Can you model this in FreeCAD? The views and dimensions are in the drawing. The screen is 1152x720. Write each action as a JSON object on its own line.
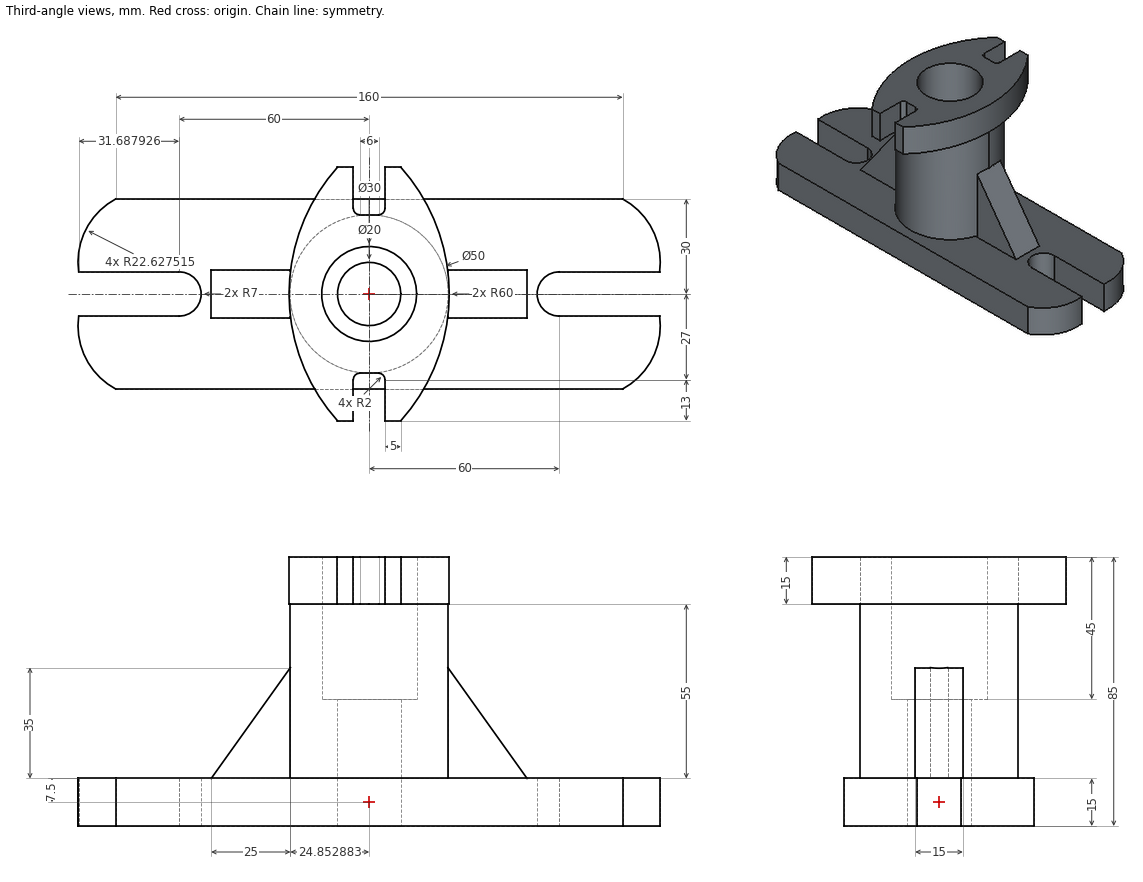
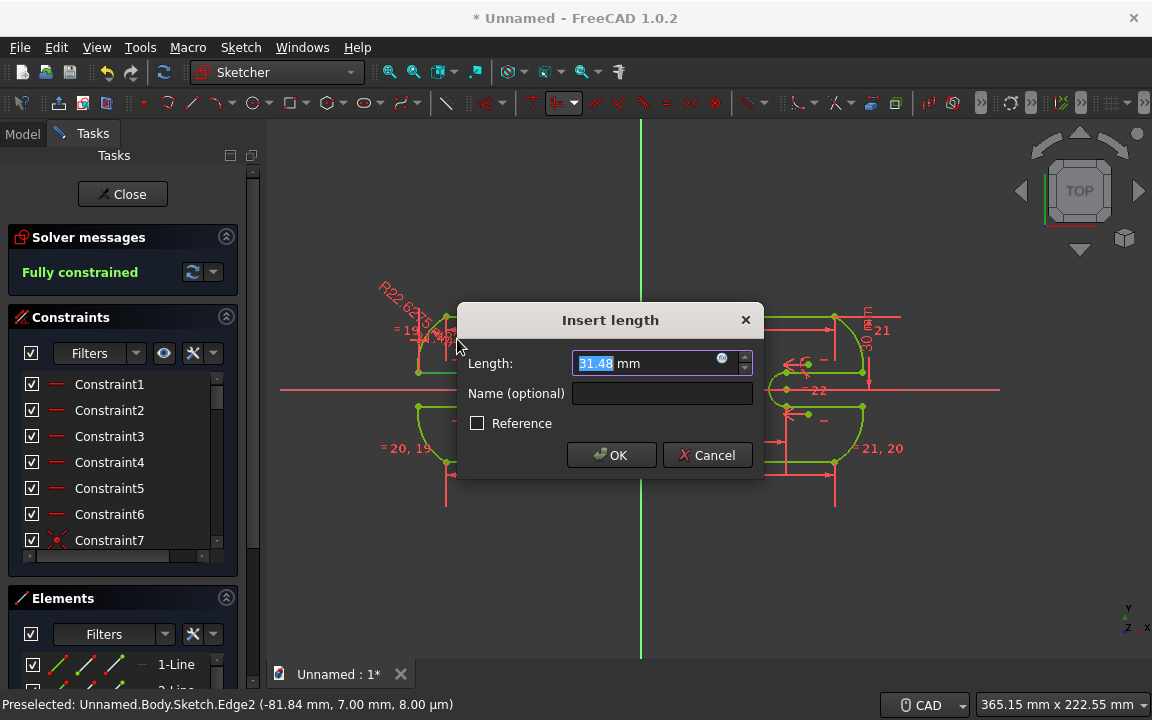
{"action": "type", "text": "31.687926"}
{"action": "key", "text": "Return"}
{"action": "key", "text": "Escape"}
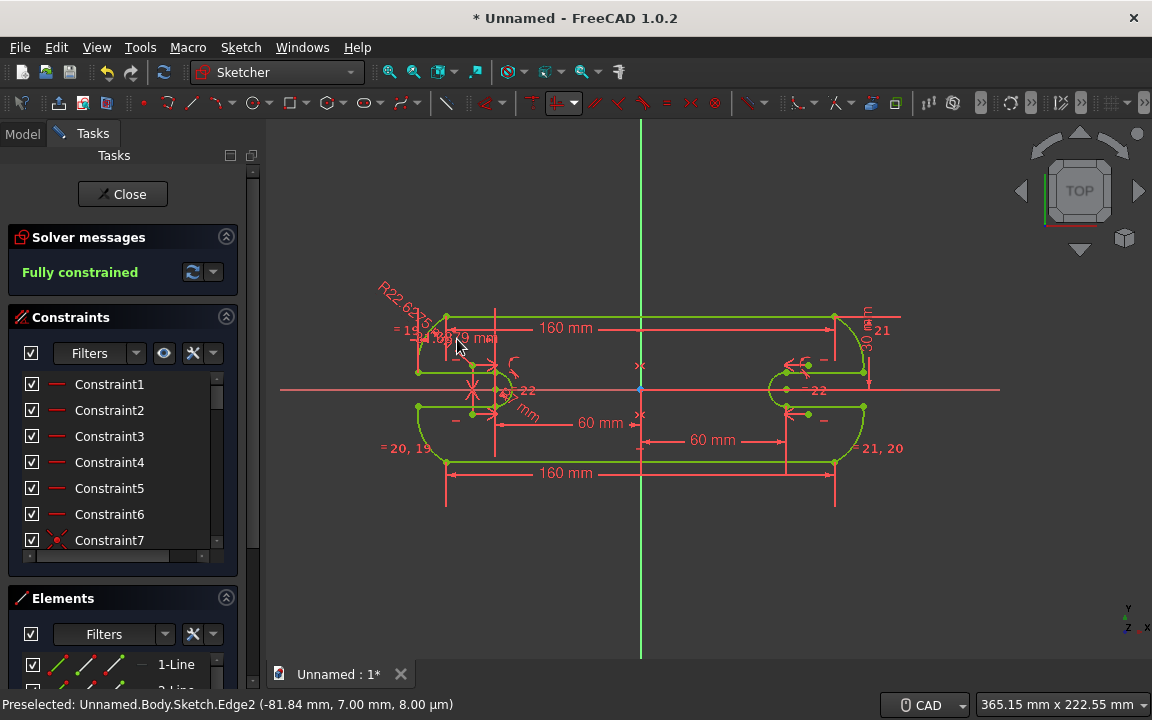
{"action": "left_click", "coordinate": [123, 194]}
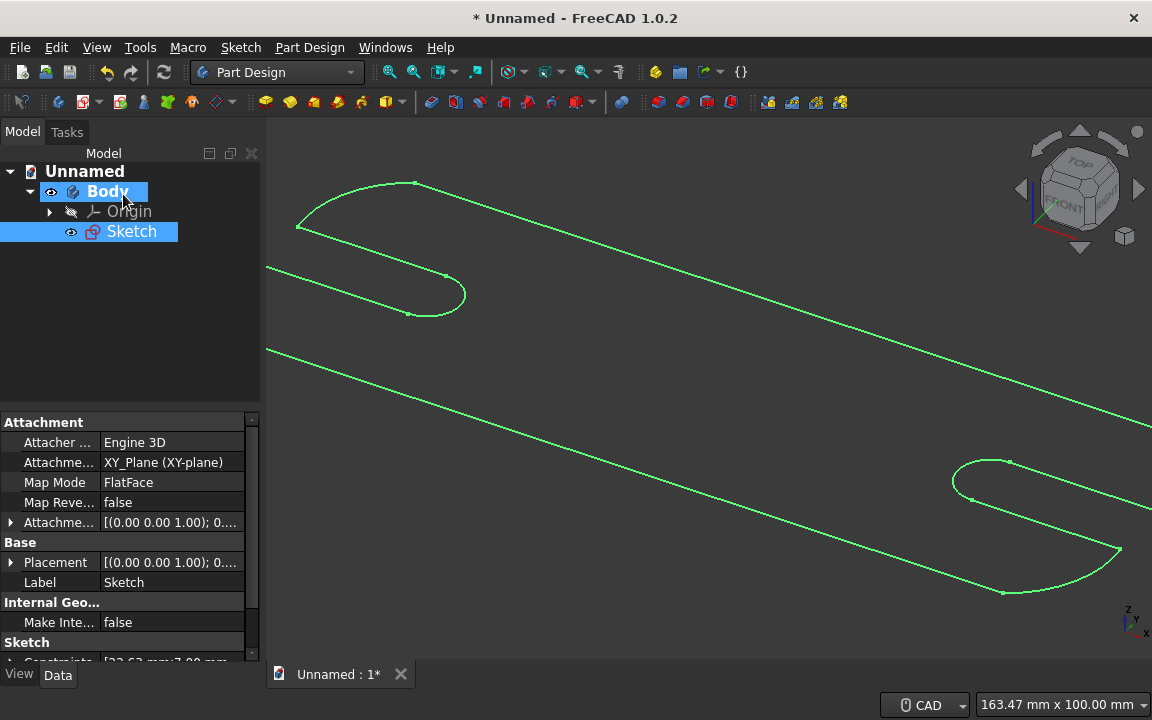
{"action": "left_click", "coordinate": [266, 102]}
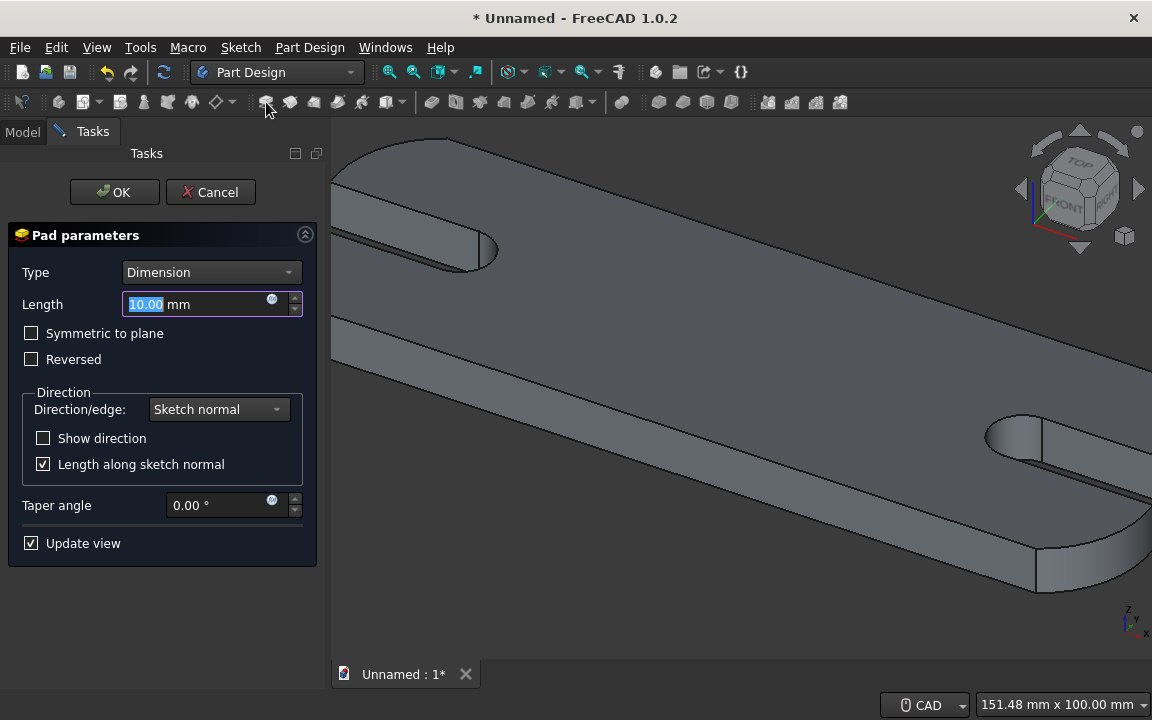
{"action": "type", "text": "15"}
{"action": "key", "text": "Tab"}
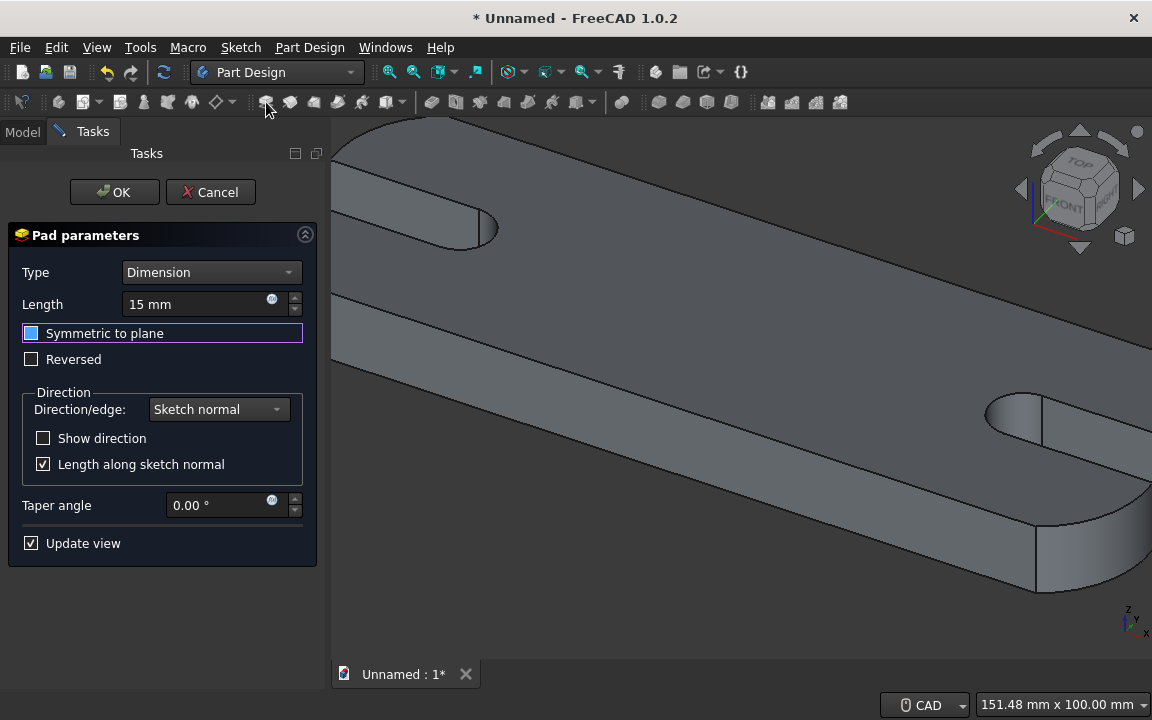
{"action": "left_click", "coordinate": [30, 333]}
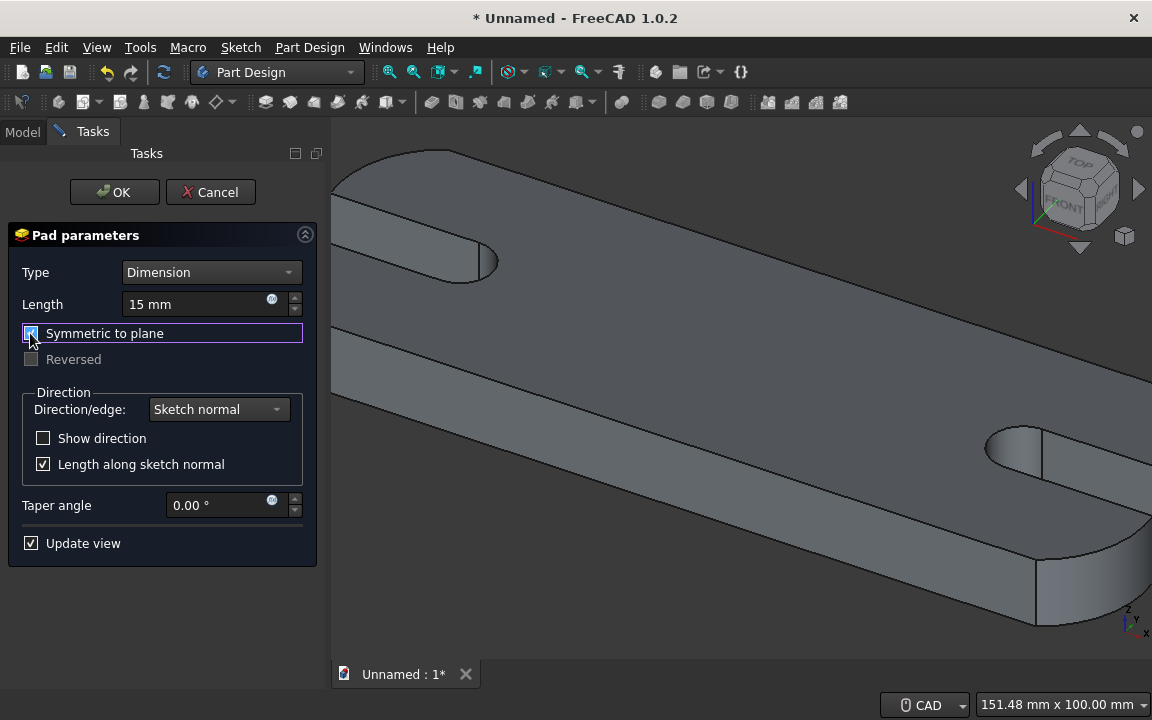
{"action": "left_click", "coordinate": [115, 192]}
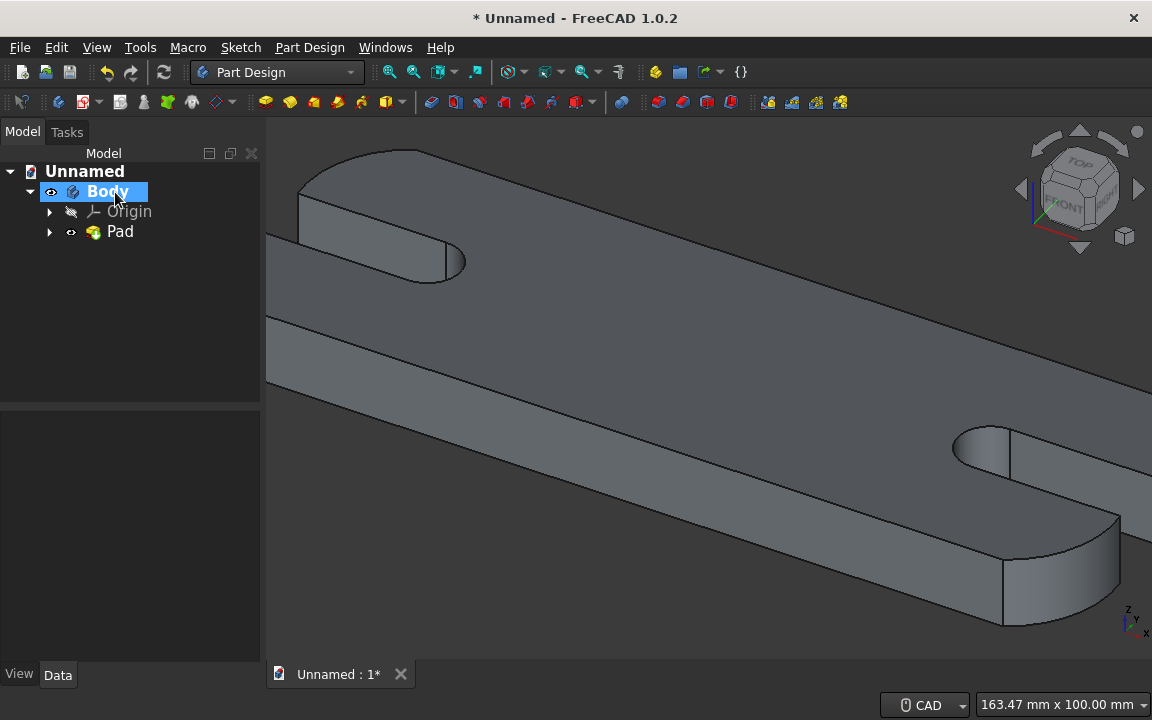
{"action": "key", "text": "v f"}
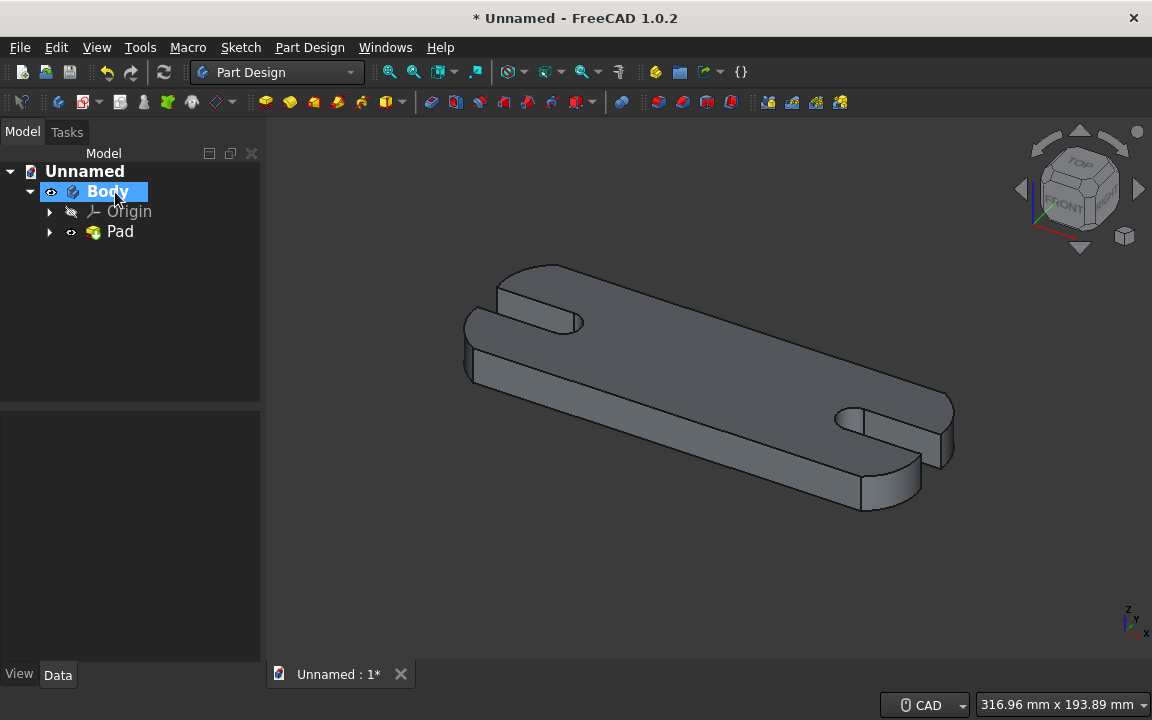
{"action": "left_click", "coordinate": [709, 370]}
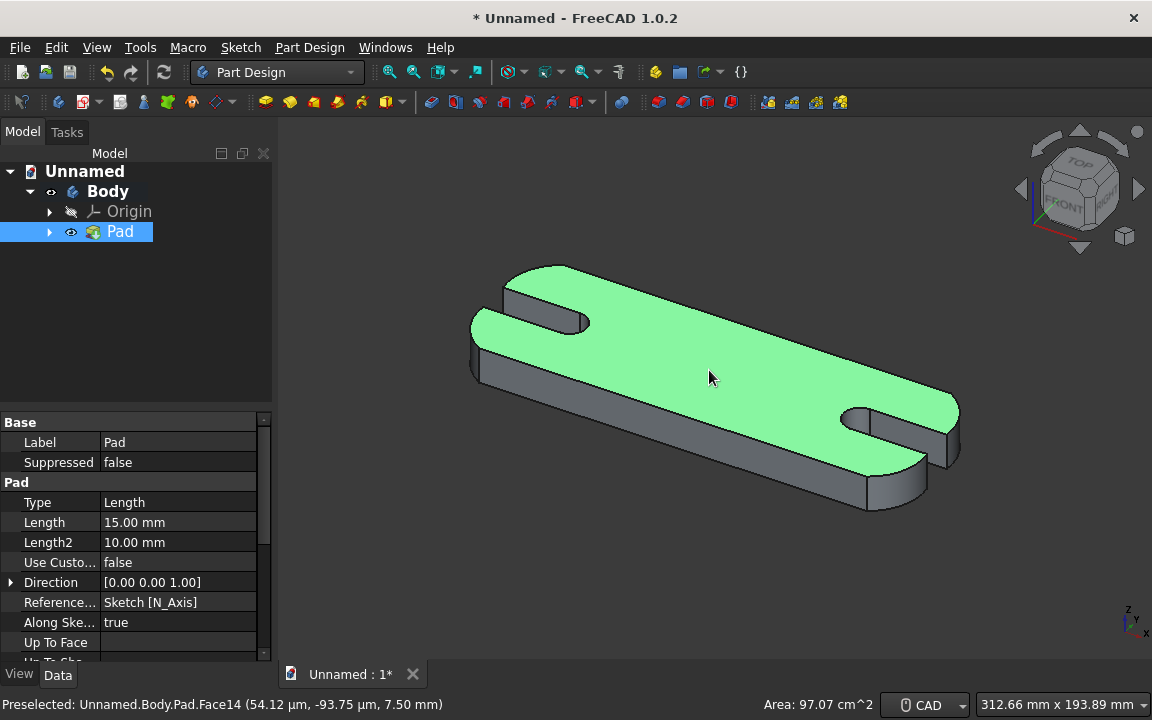
{"action": "left_click", "coordinate": [84, 102]}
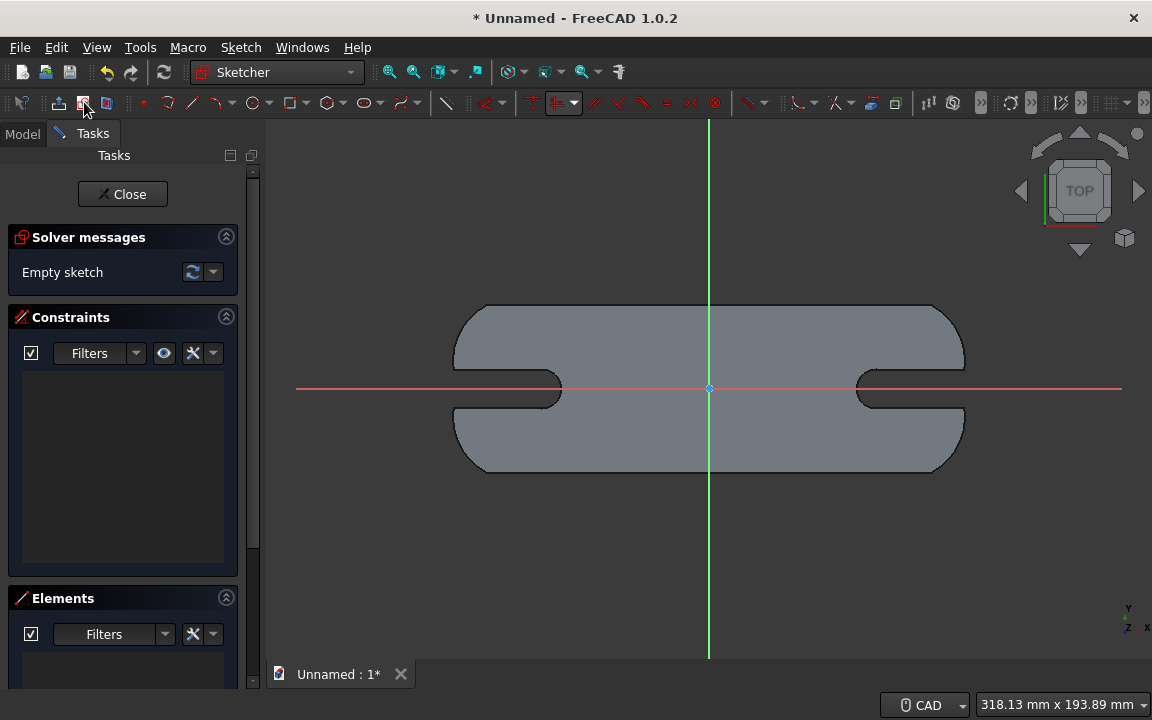
{"action": "scroll", "coordinate": [765, 389], "scroll_direction": "up", "scroll_amount": 4}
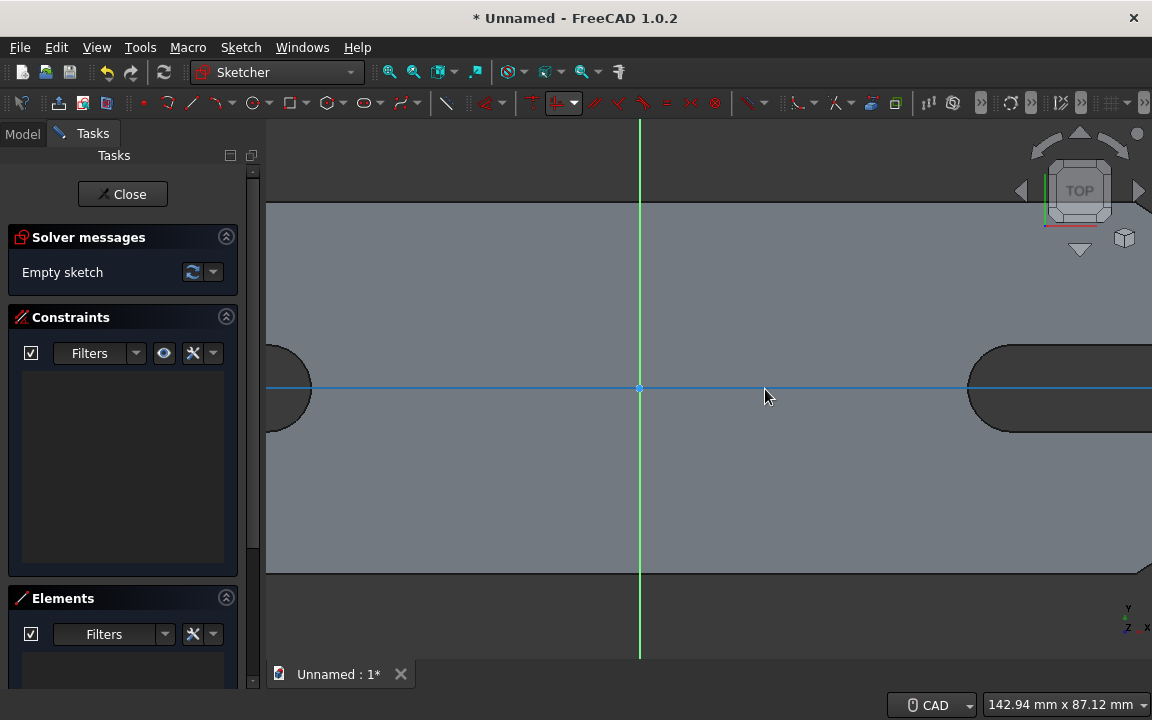
{"action": "key", "text": "g c"}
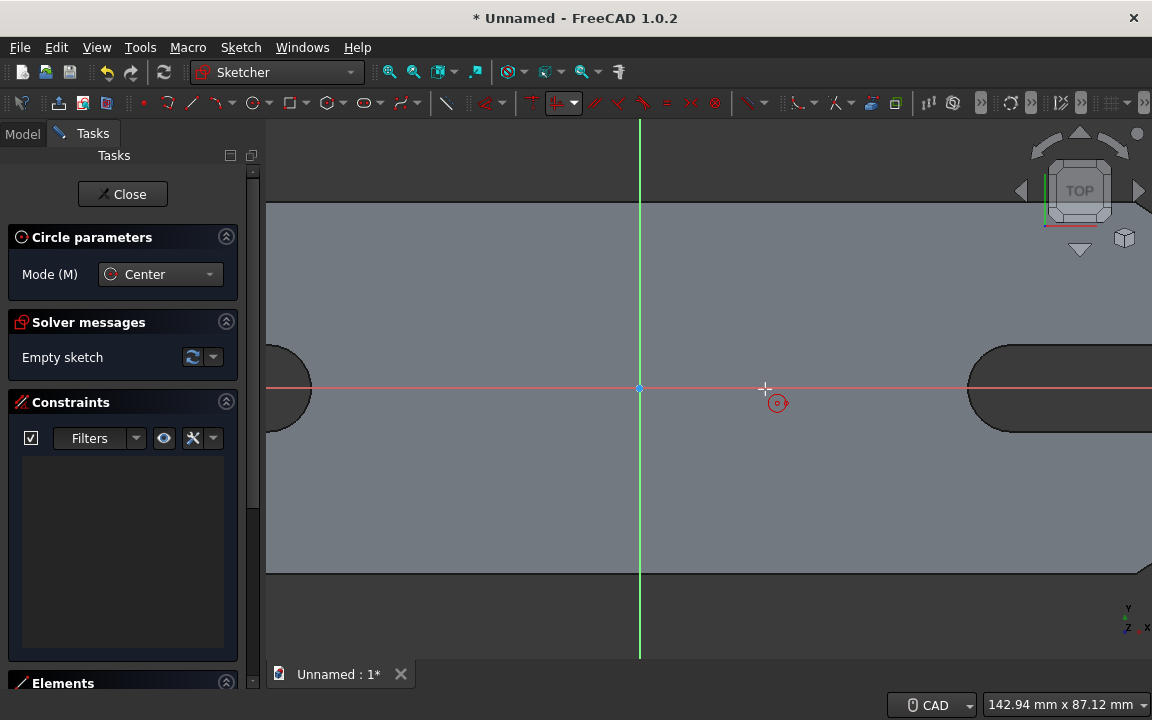
{"action": "left_click", "coordinate": [640, 388]}
{"action": "mouse_move", "coordinate": [749, 279]}